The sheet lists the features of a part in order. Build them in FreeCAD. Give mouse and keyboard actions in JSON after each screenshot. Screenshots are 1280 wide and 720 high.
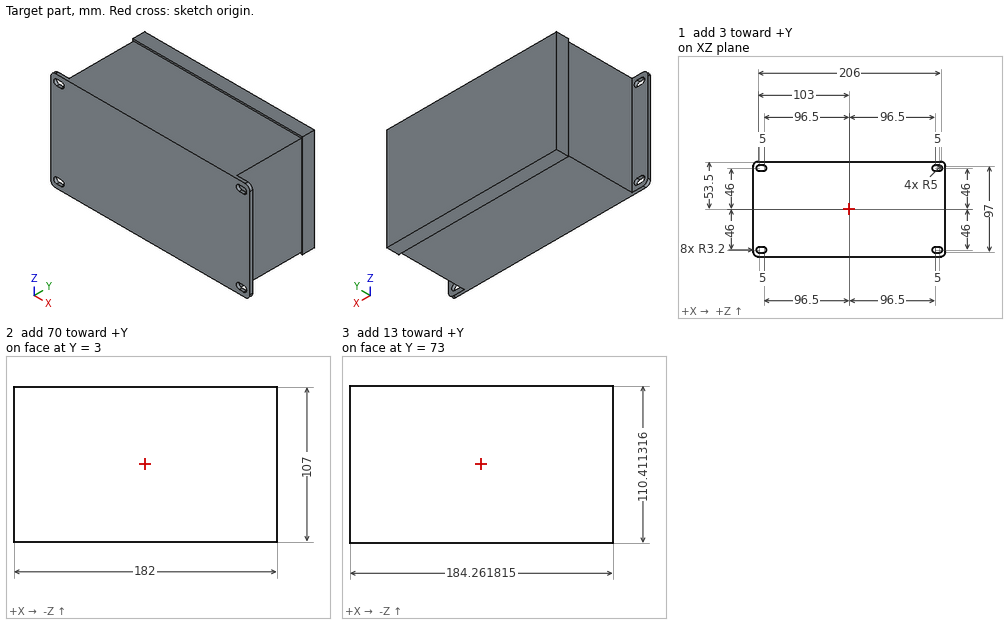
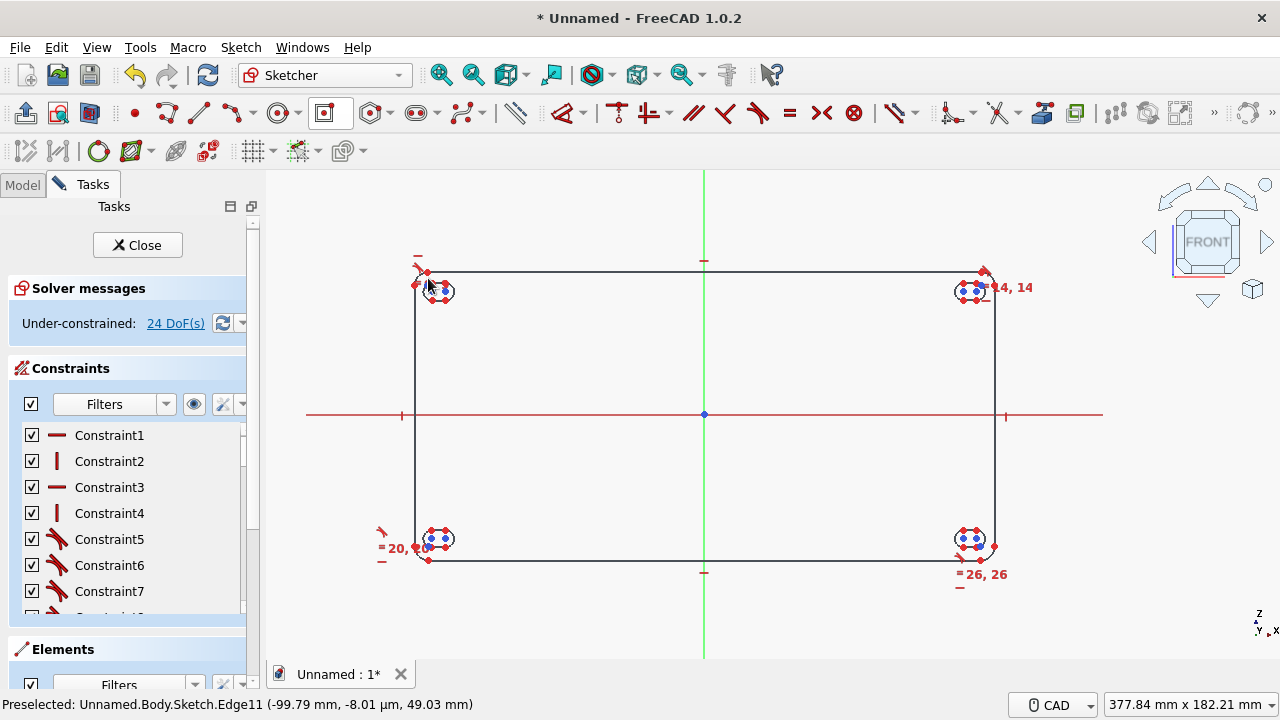
{"action": "scroll", "coordinate": [993, 280], "scroll_direction": "up", "scroll_amount": 5}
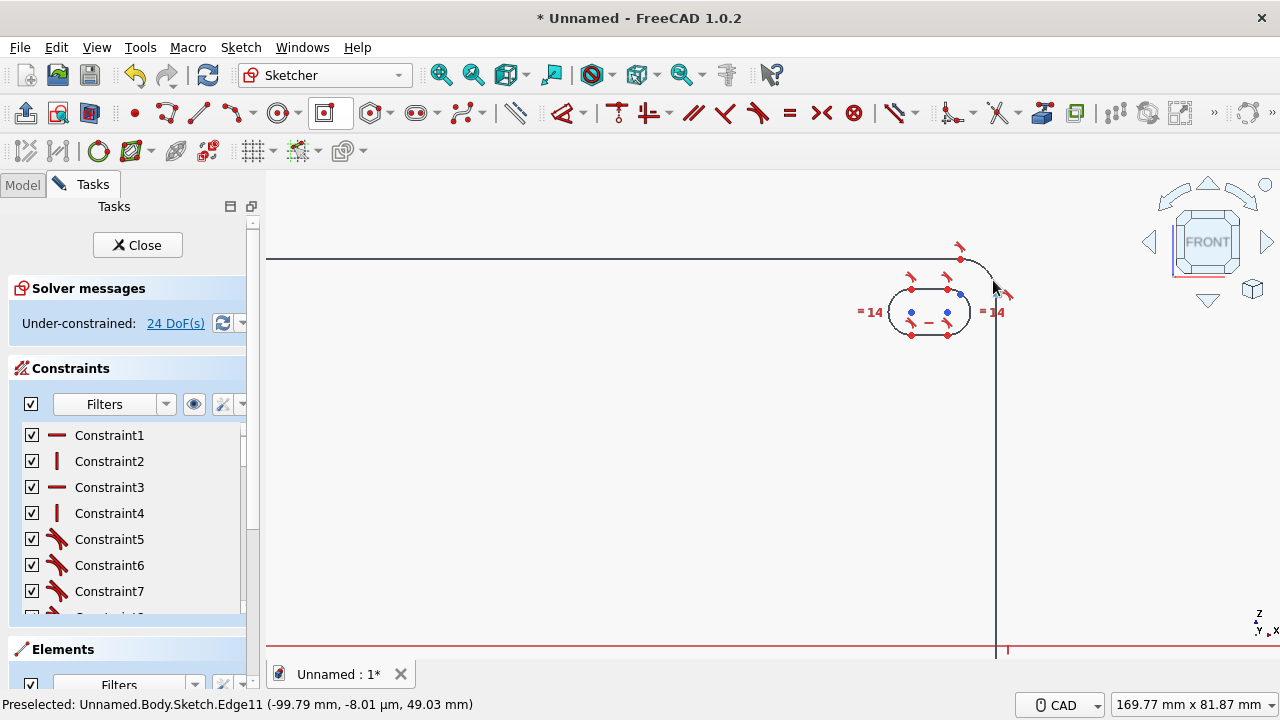
{"action": "left_click", "coordinate": [992, 278]}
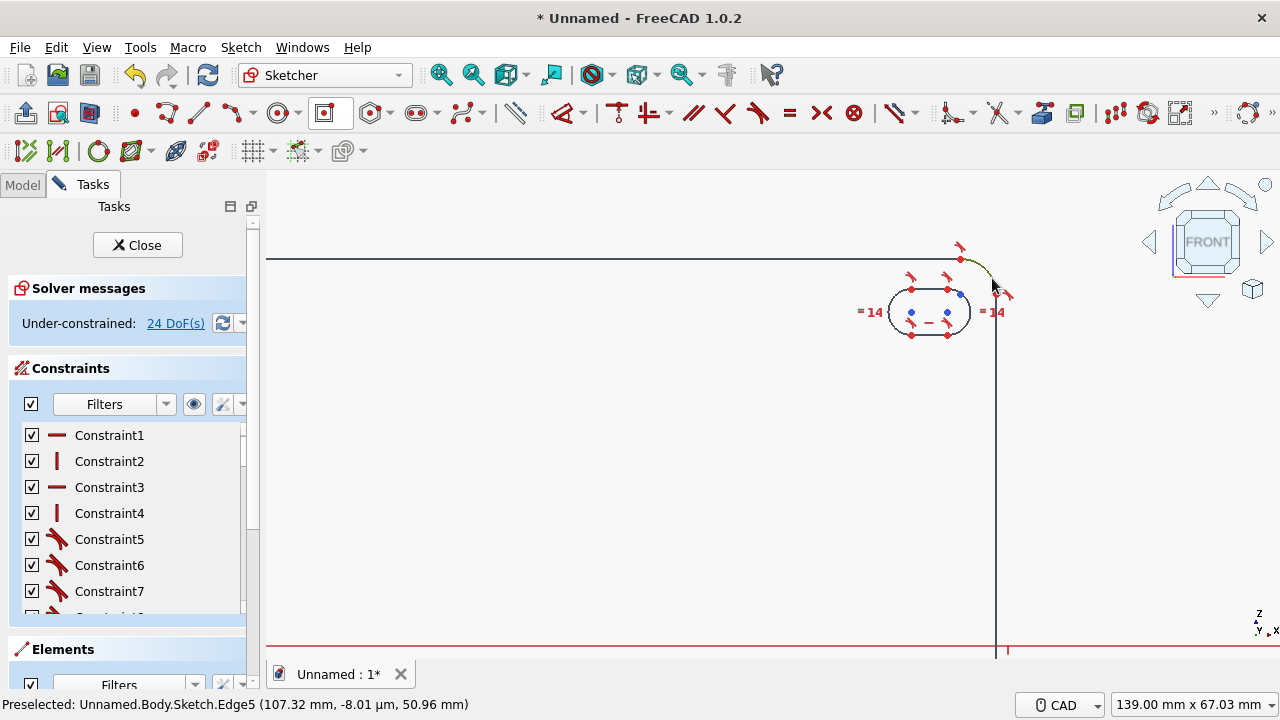
{"action": "scroll", "coordinate": [994, 280], "scroll_direction": "down", "scroll_amount": 5}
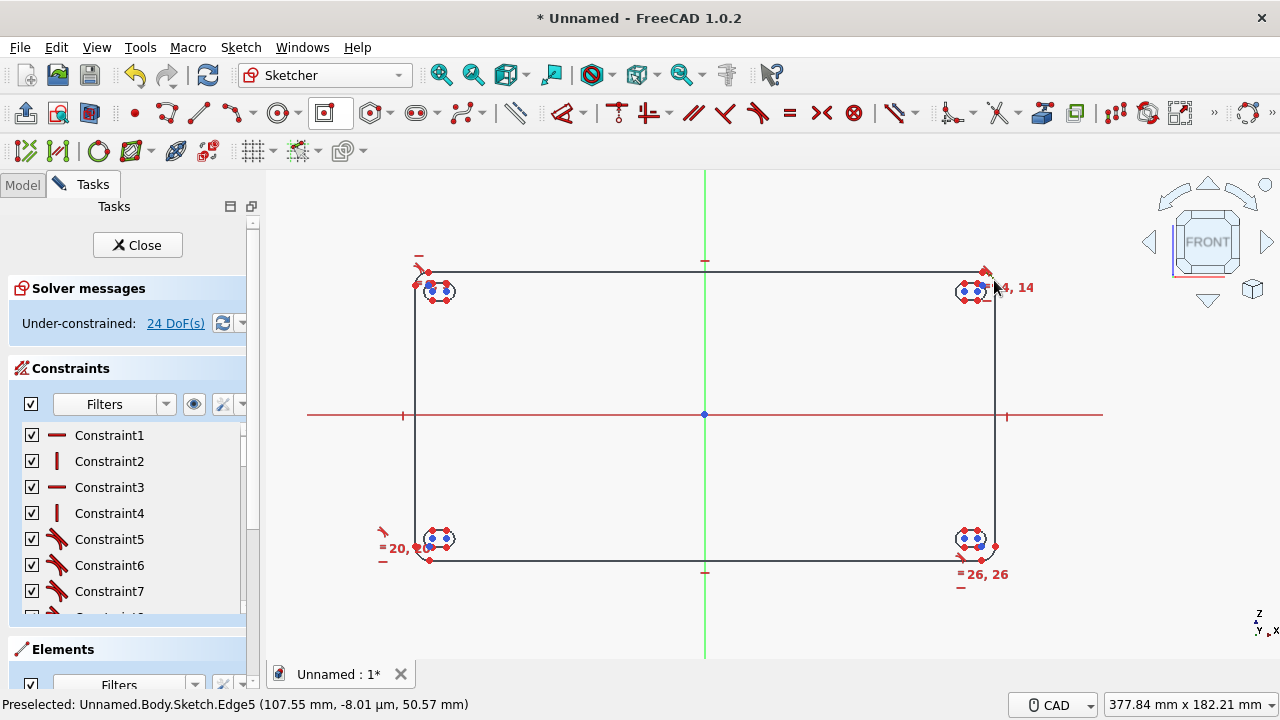
{"action": "scroll", "coordinate": [988, 559], "scroll_direction": "up", "scroll_amount": 4}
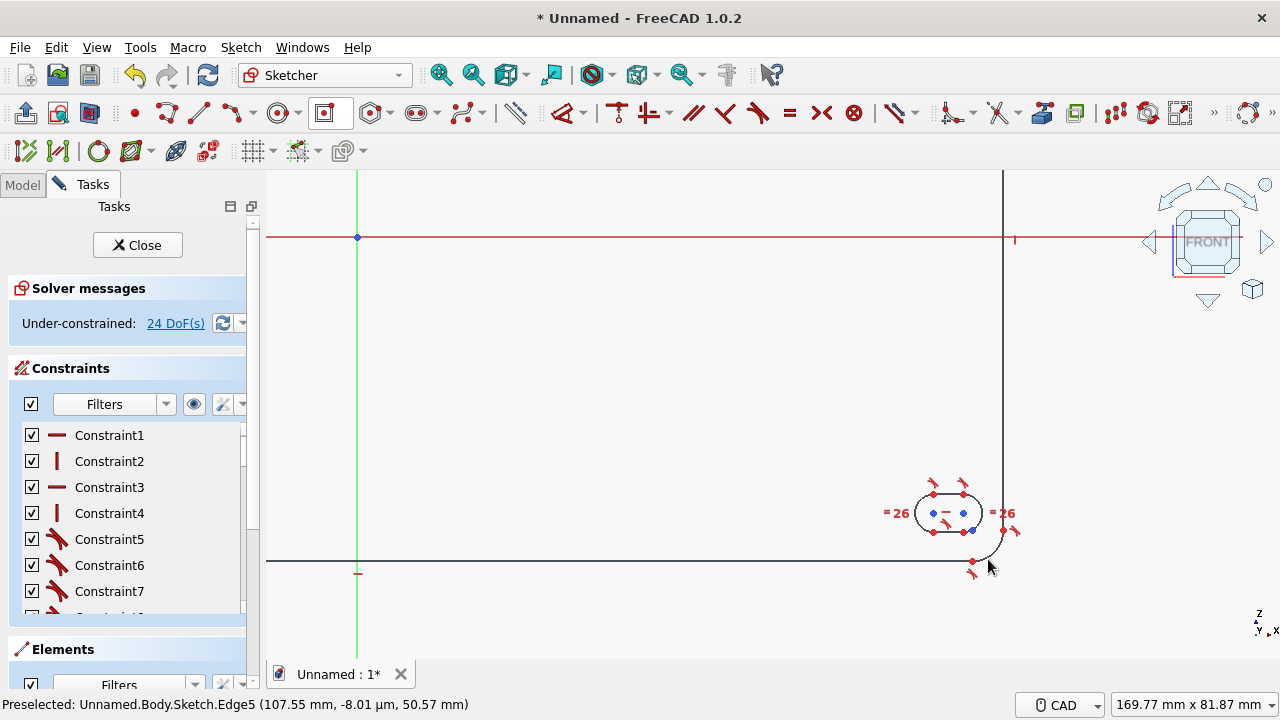
{"action": "left_click", "coordinate": [986, 558]}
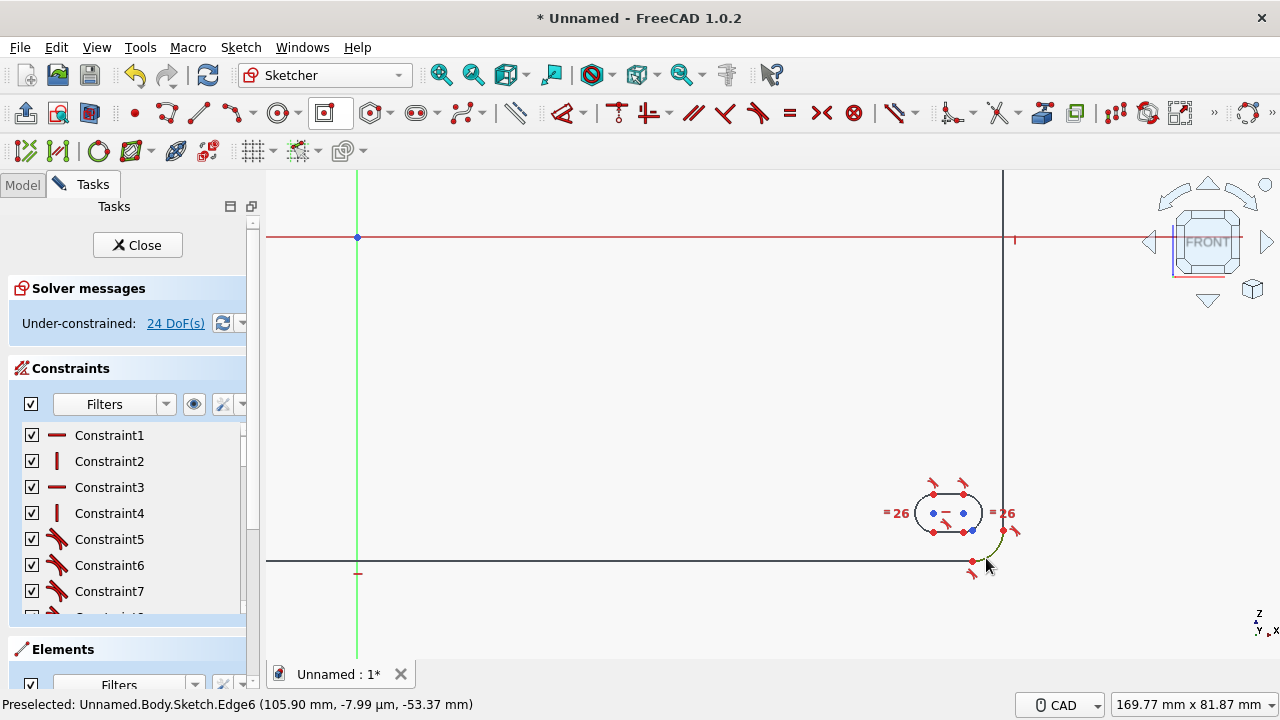
{"action": "scroll", "coordinate": [988, 559], "scroll_direction": "down", "scroll_amount": 4}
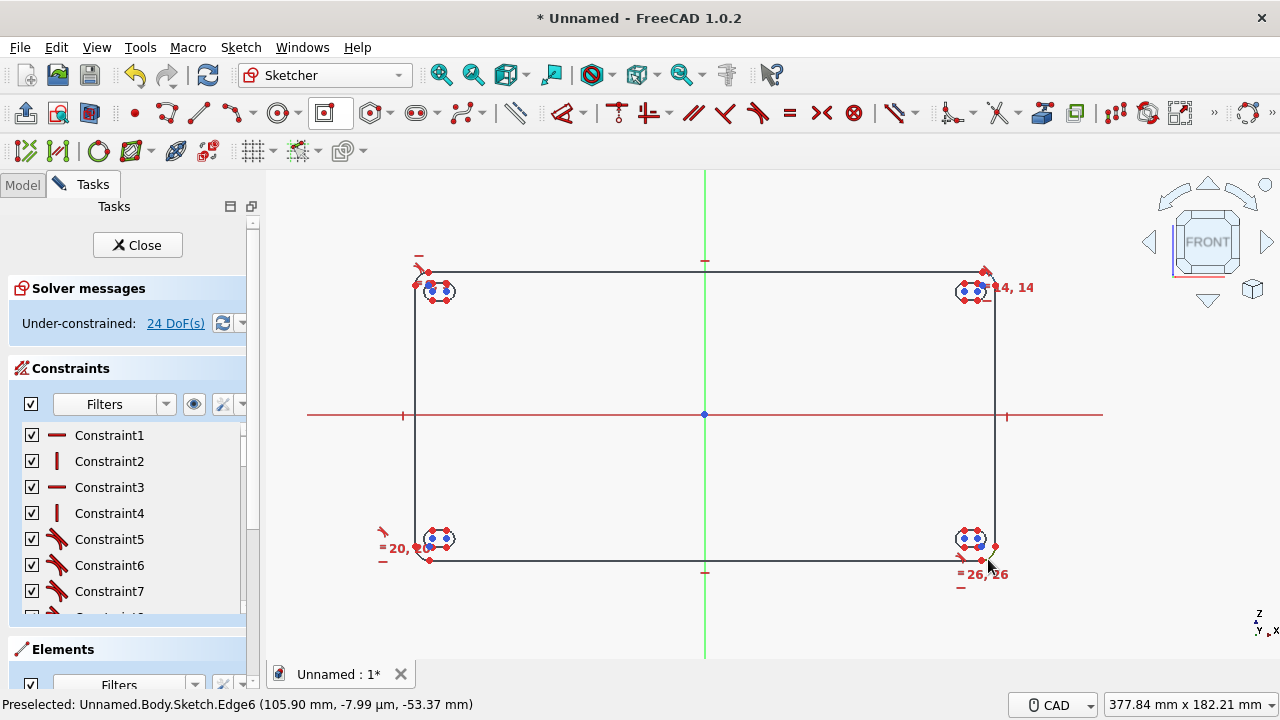
{"action": "scroll", "coordinate": [417, 553], "scroll_direction": "up", "scroll_amount": 4}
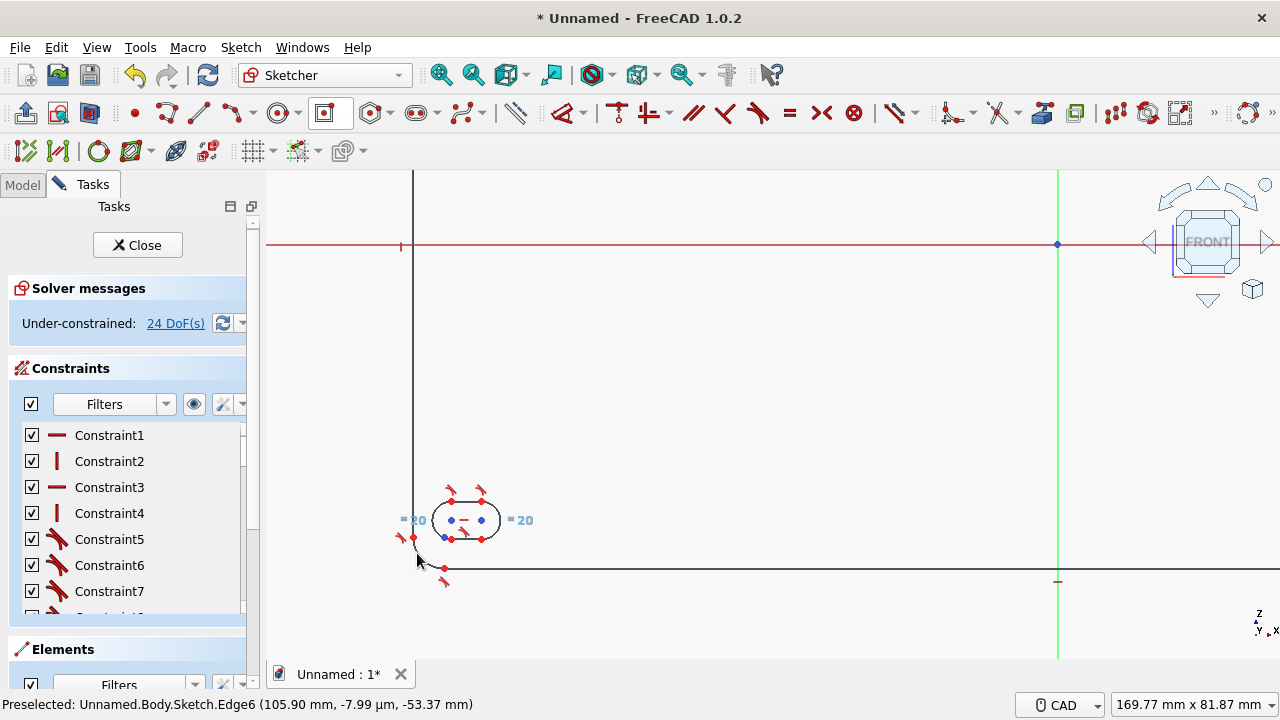
{"action": "left_click", "coordinate": [417, 552]}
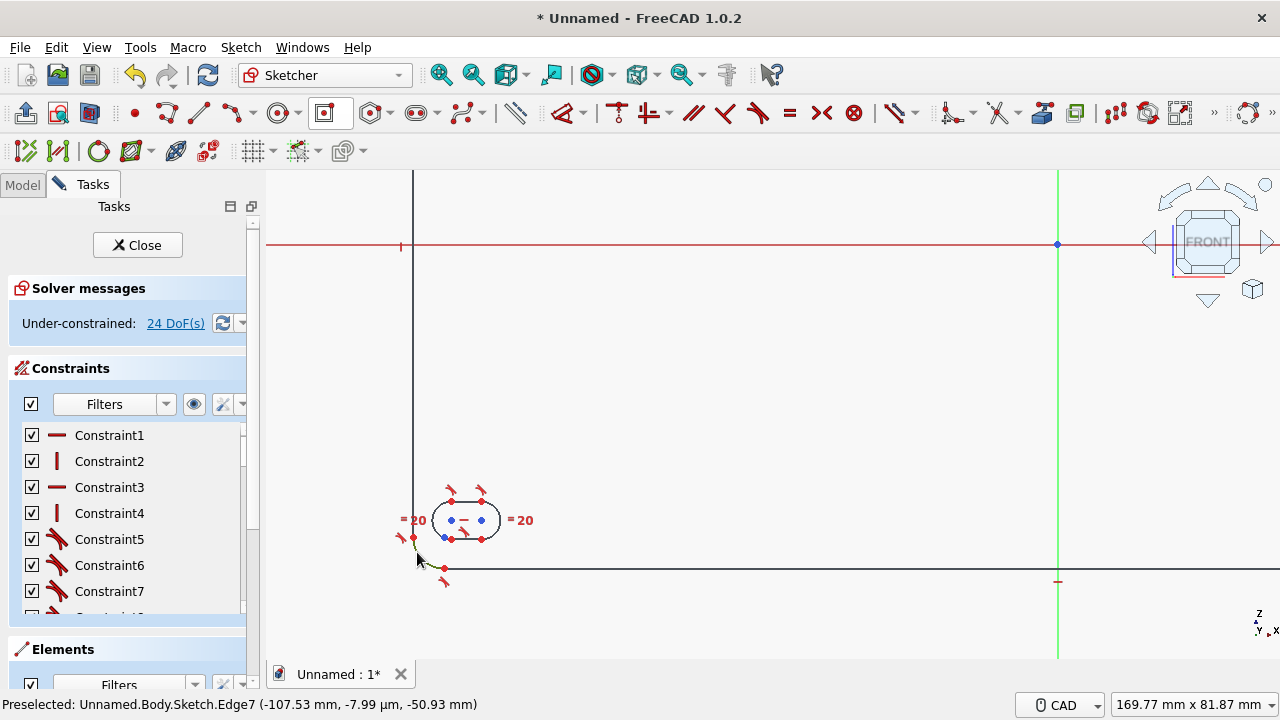
{"action": "scroll", "coordinate": [416, 553], "scroll_direction": "down", "scroll_amount": 4}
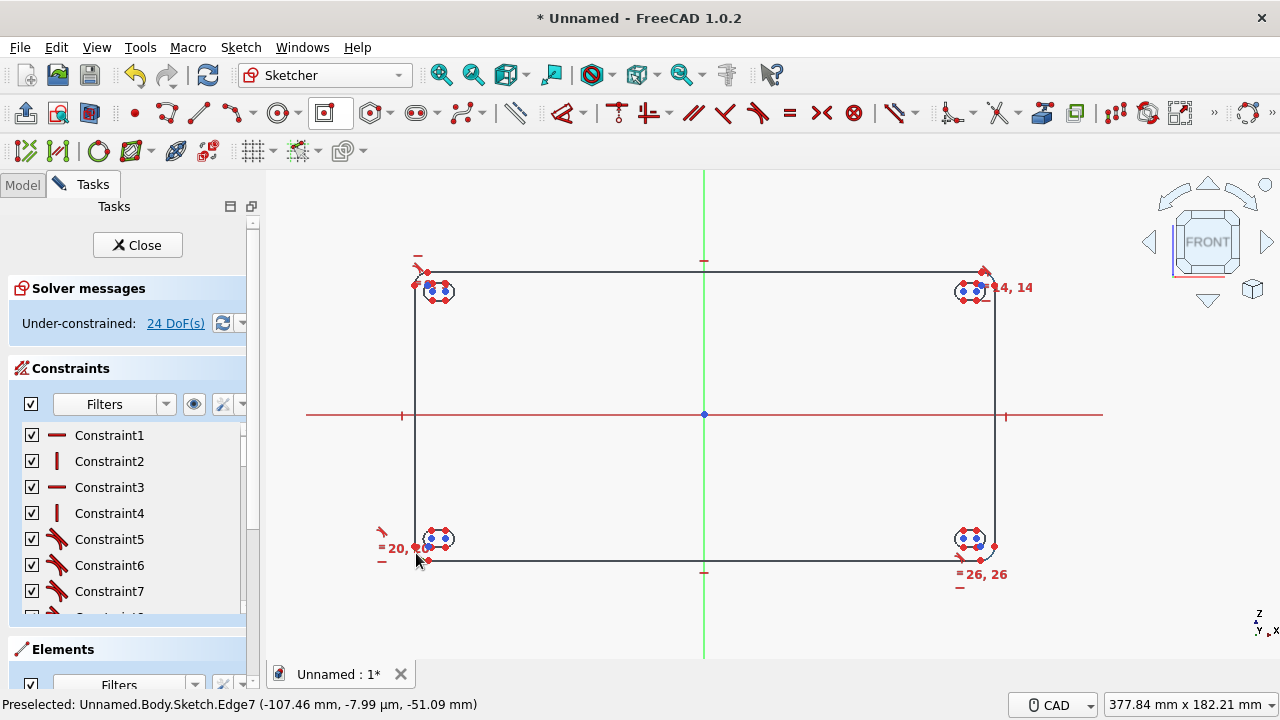
{"action": "scroll", "coordinate": [422, 274], "scroll_direction": "up", "scroll_amount": 5}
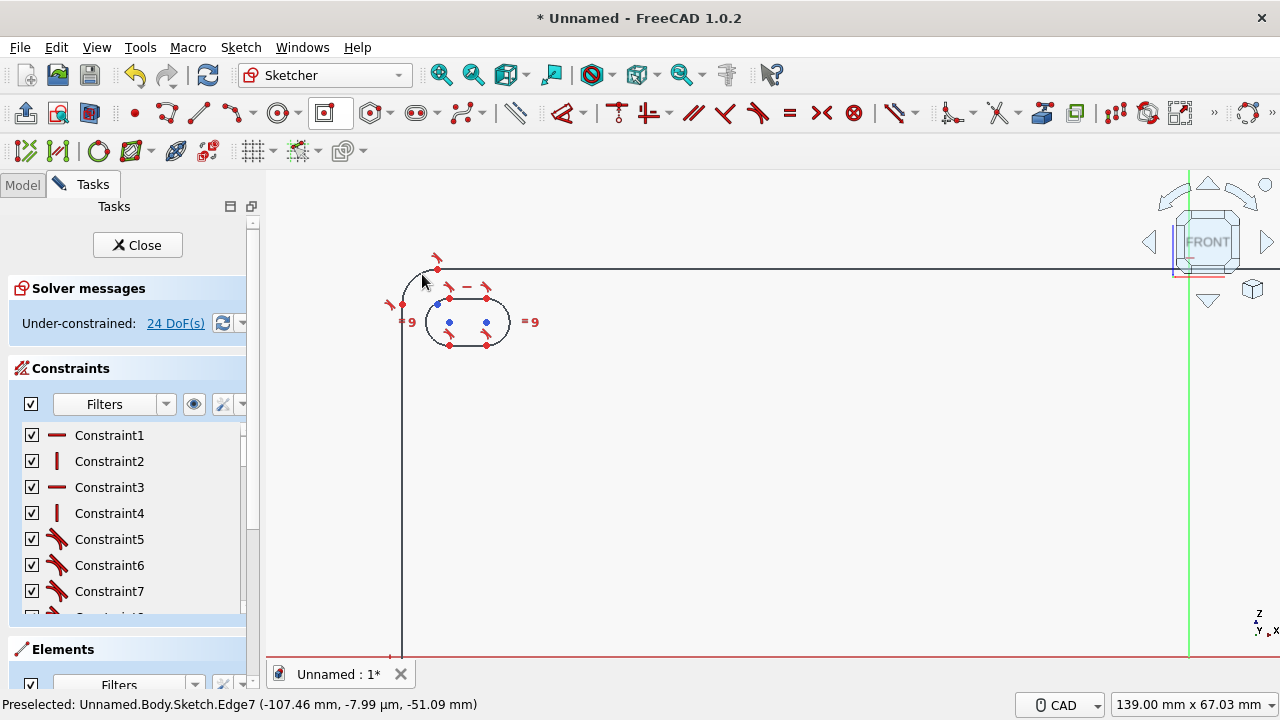
{"action": "left_click", "coordinate": [422, 273]}